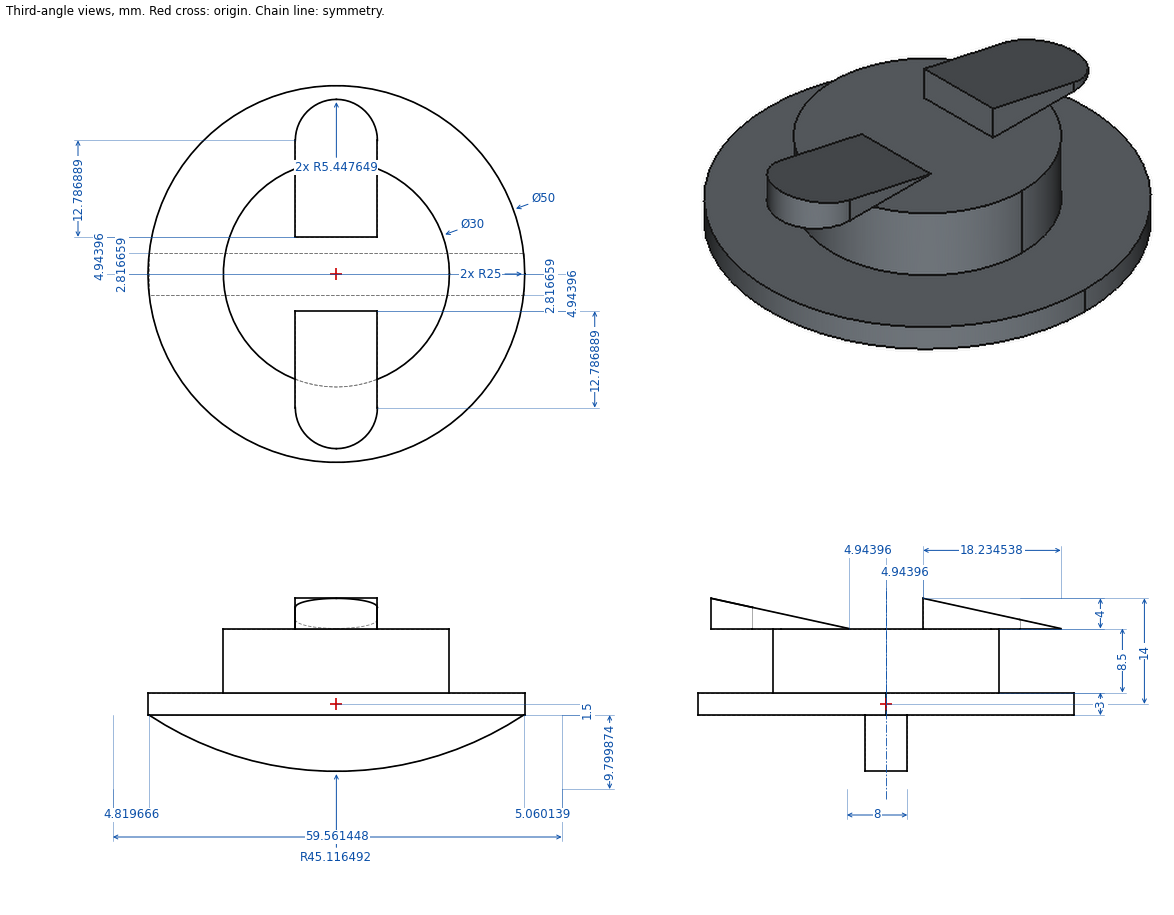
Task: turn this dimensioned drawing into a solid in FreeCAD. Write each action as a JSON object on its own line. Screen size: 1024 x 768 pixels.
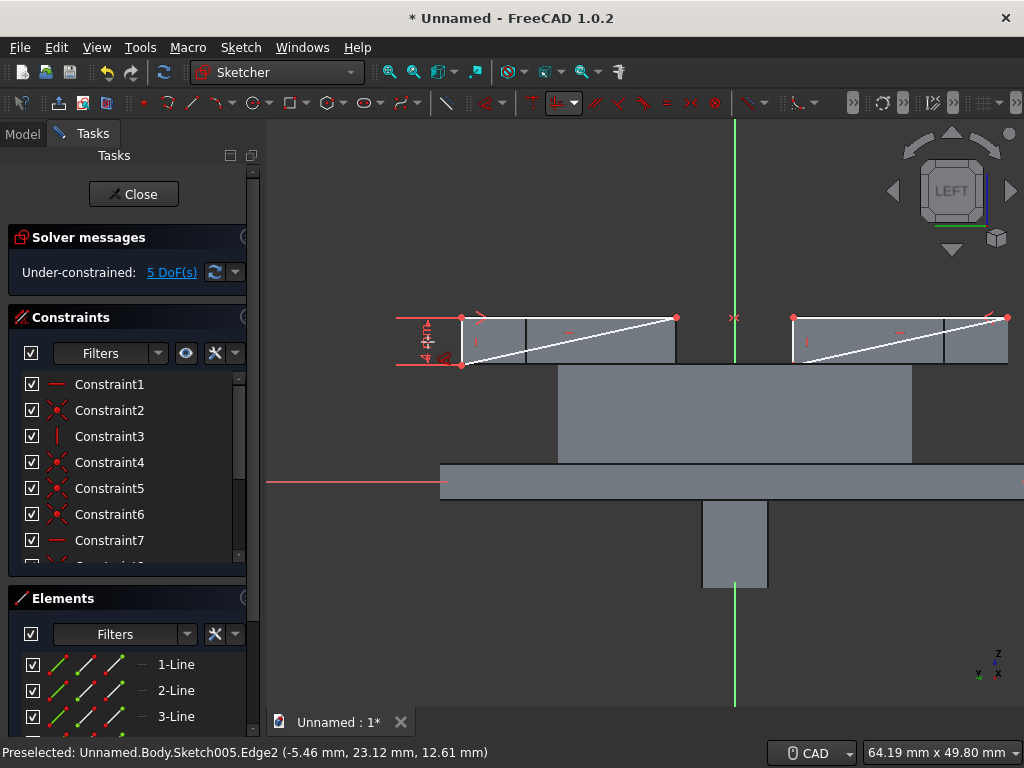
{"action": "left_click", "coordinate": [793, 332]}
{"action": "left_click", "coordinate": [827, 342]}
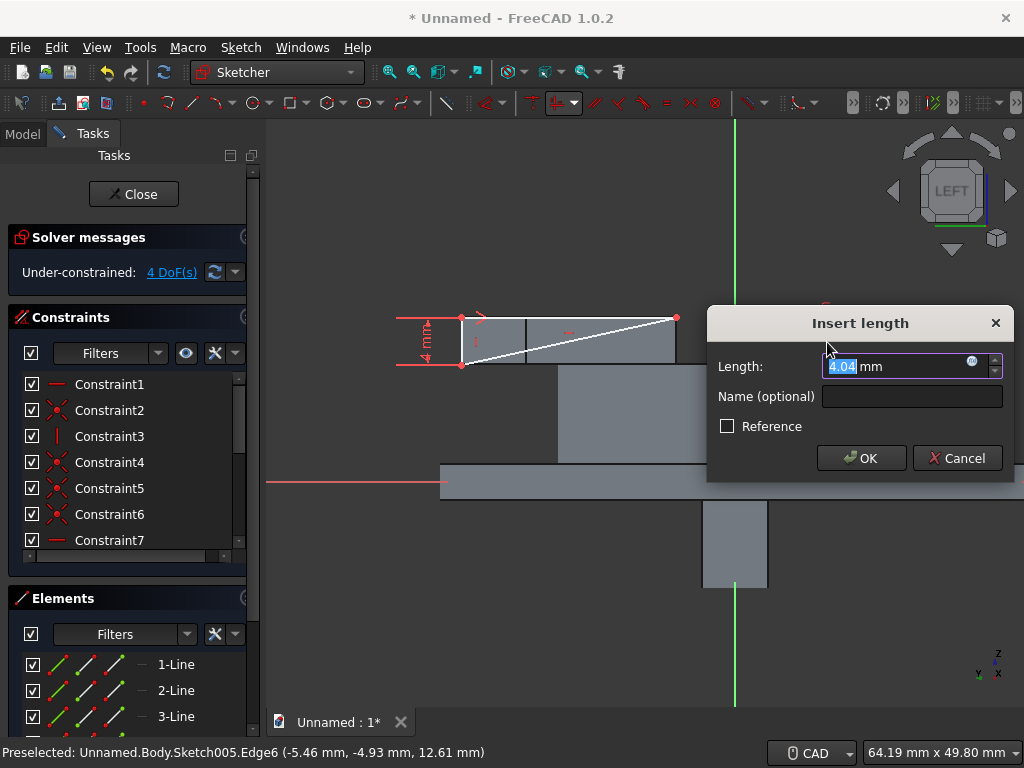
{"action": "type", "text": "4"}
{"action": "key", "text": "Return"}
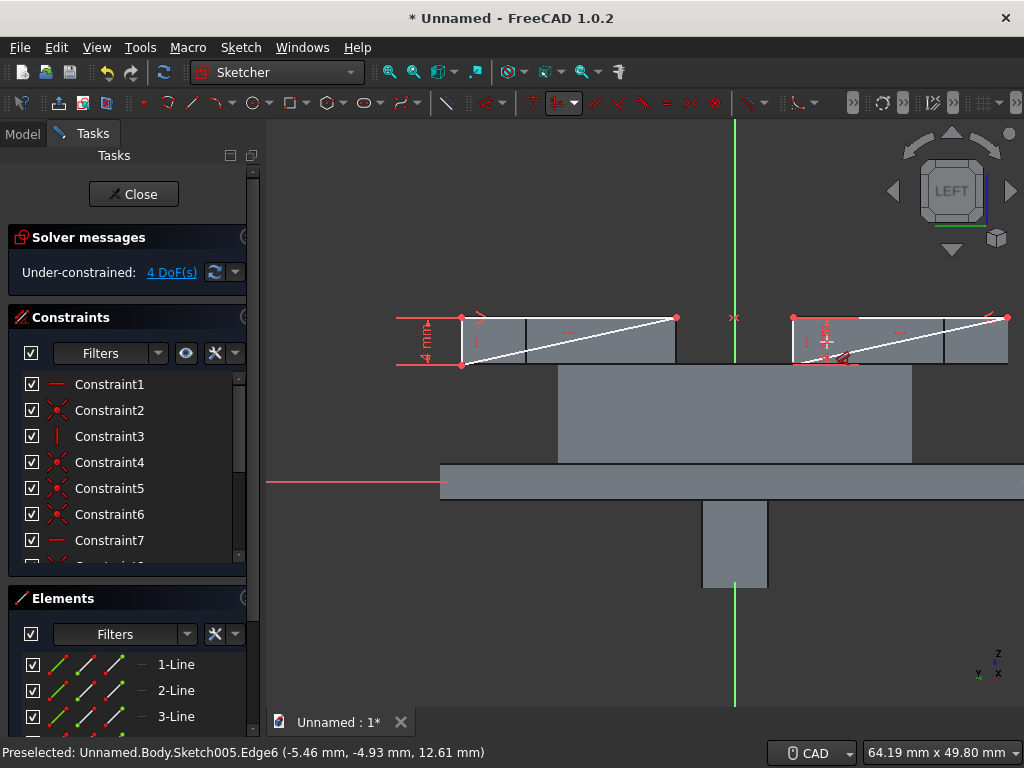
{"action": "left_click", "coordinate": [677, 318]}
{"action": "left_click", "coordinate": [643, 400]}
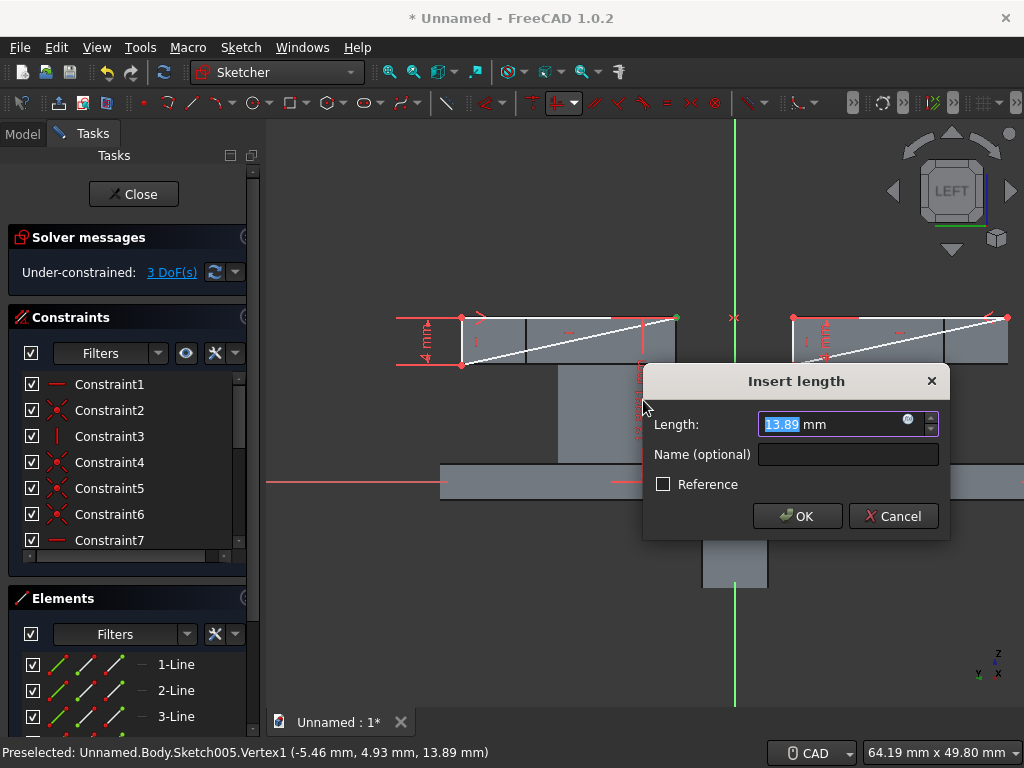
{"action": "type", "text": "14"}
{"action": "key", "text": "Return"}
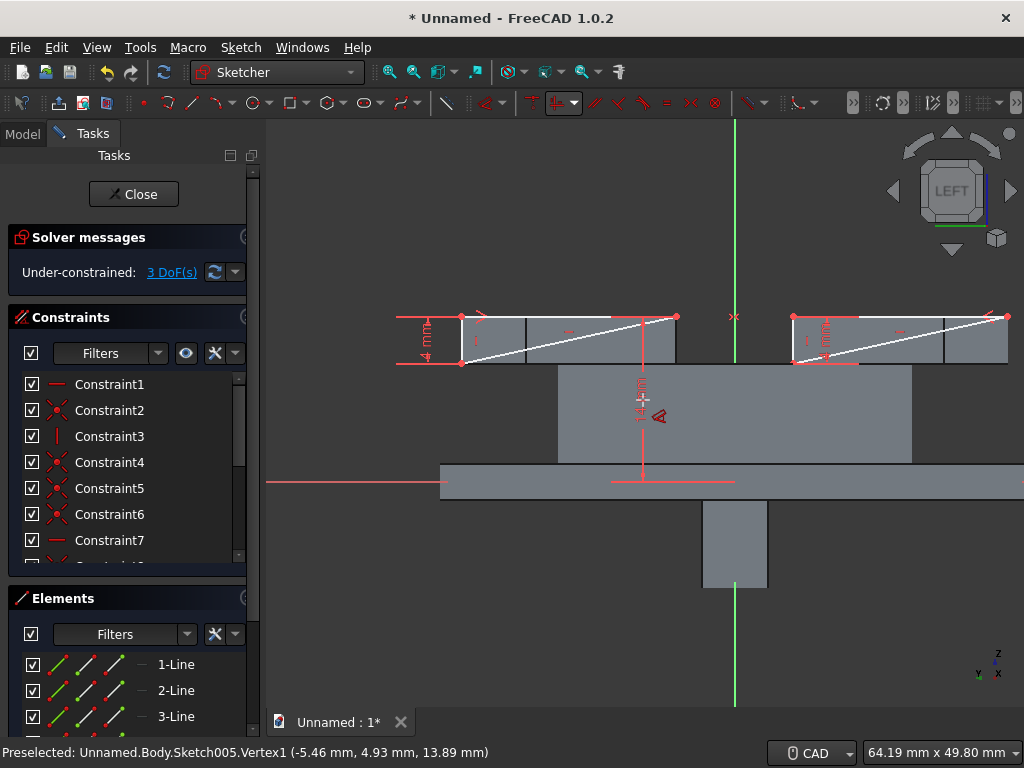
{"action": "left_click", "coordinate": [677, 317]}
{"action": "left_click", "coordinate": [706, 516]}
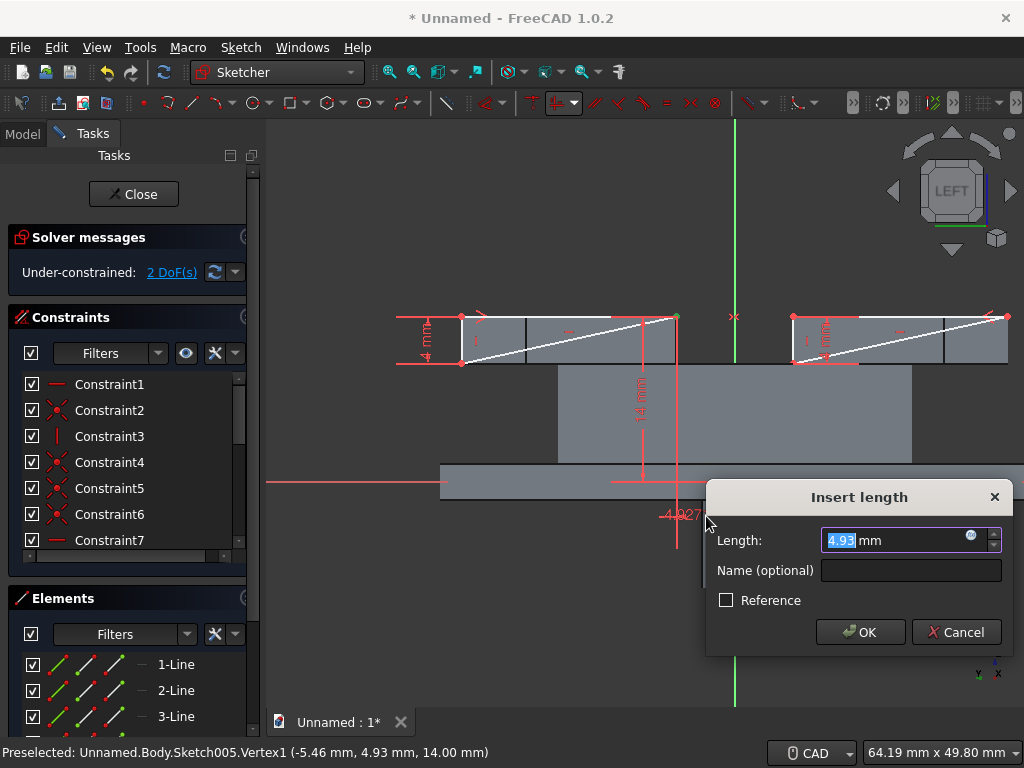
{"action": "type", "text": "4.94396"}
{"action": "key", "text": "Return"}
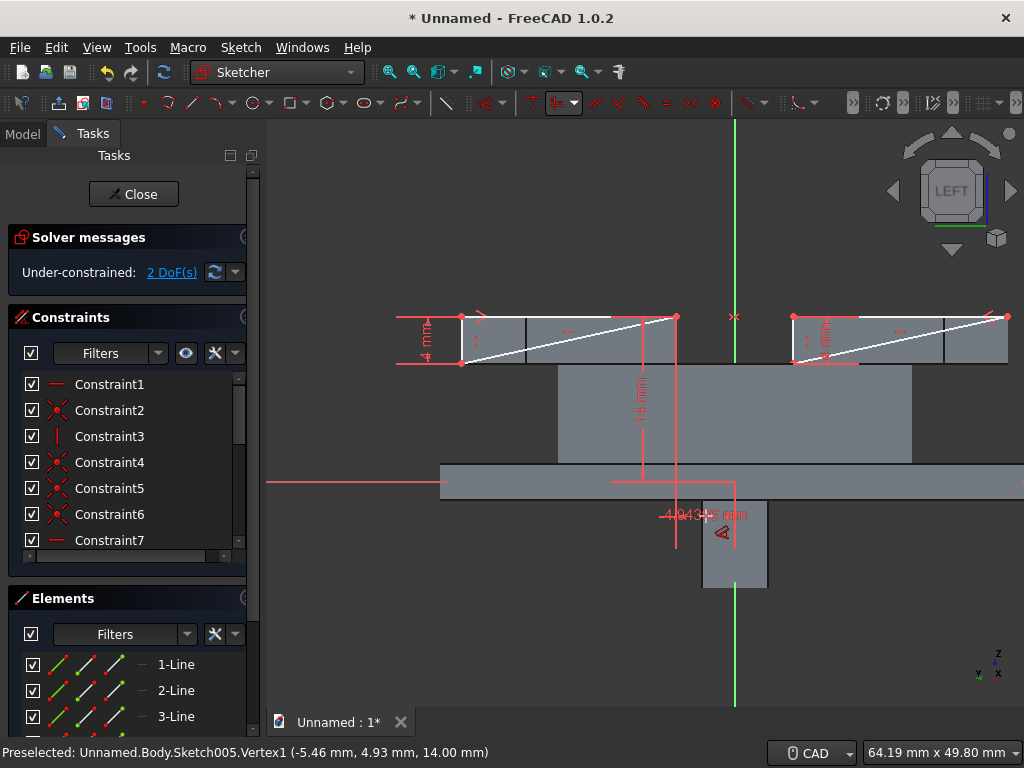
{"action": "left_click", "coordinate": [793, 364]}
{"action": "left_click", "coordinate": [777, 516]}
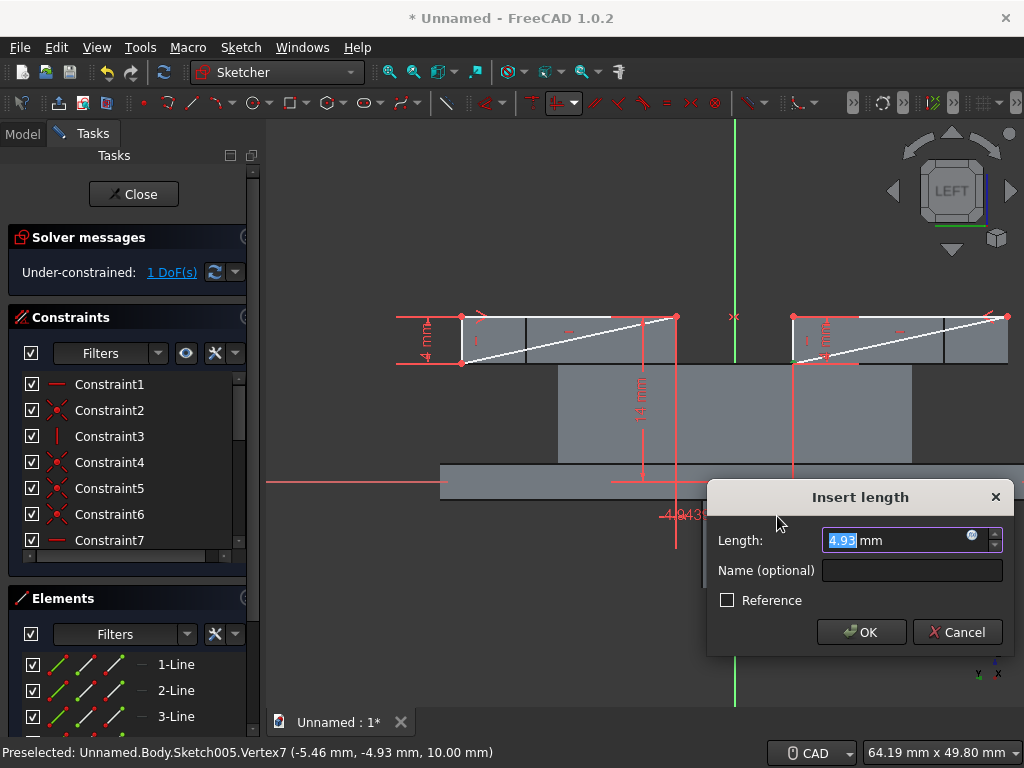
{"action": "type", "text": "4.94396"}
{"action": "key", "text": "Return"}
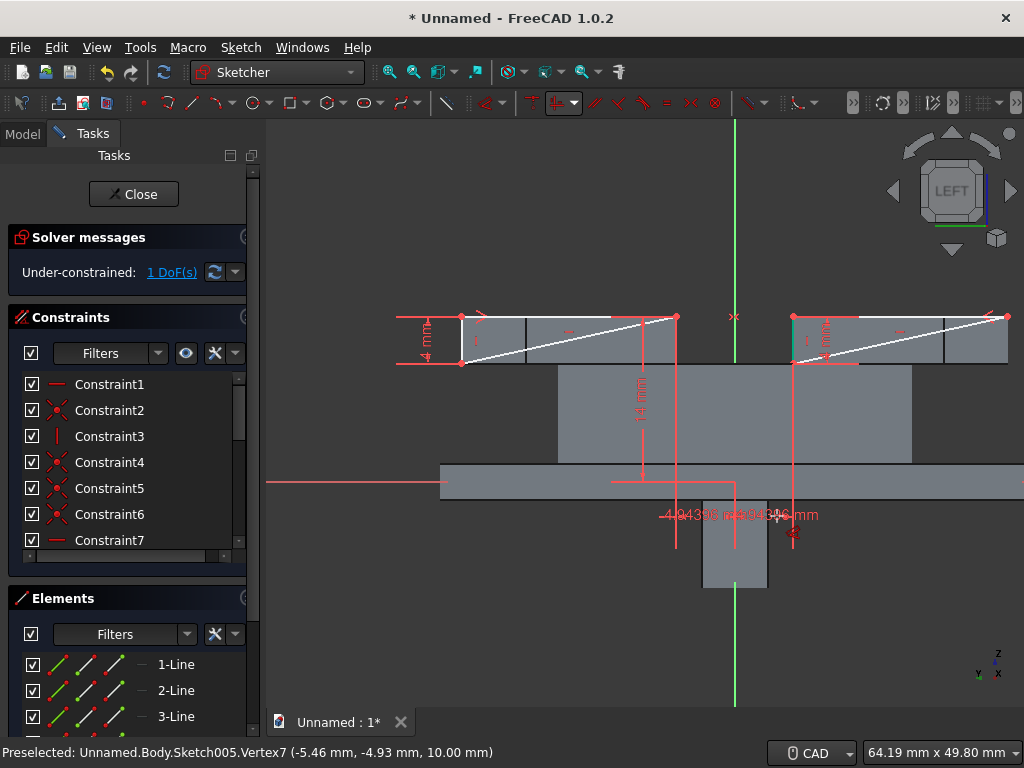
{"action": "left_click", "coordinate": [612, 317]}
{"action": "left_click", "coordinate": [569, 283]}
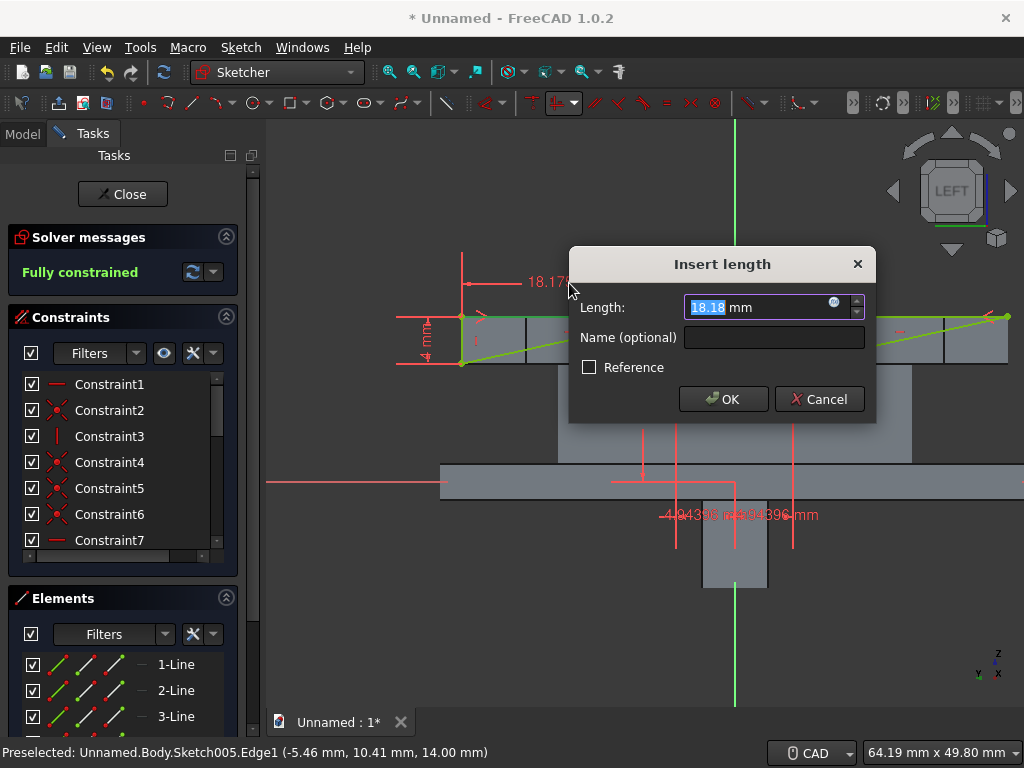
{"action": "type", "text": "18.234538"}
{"action": "key", "text": "Return"}
{"action": "key", "text": "Escape"}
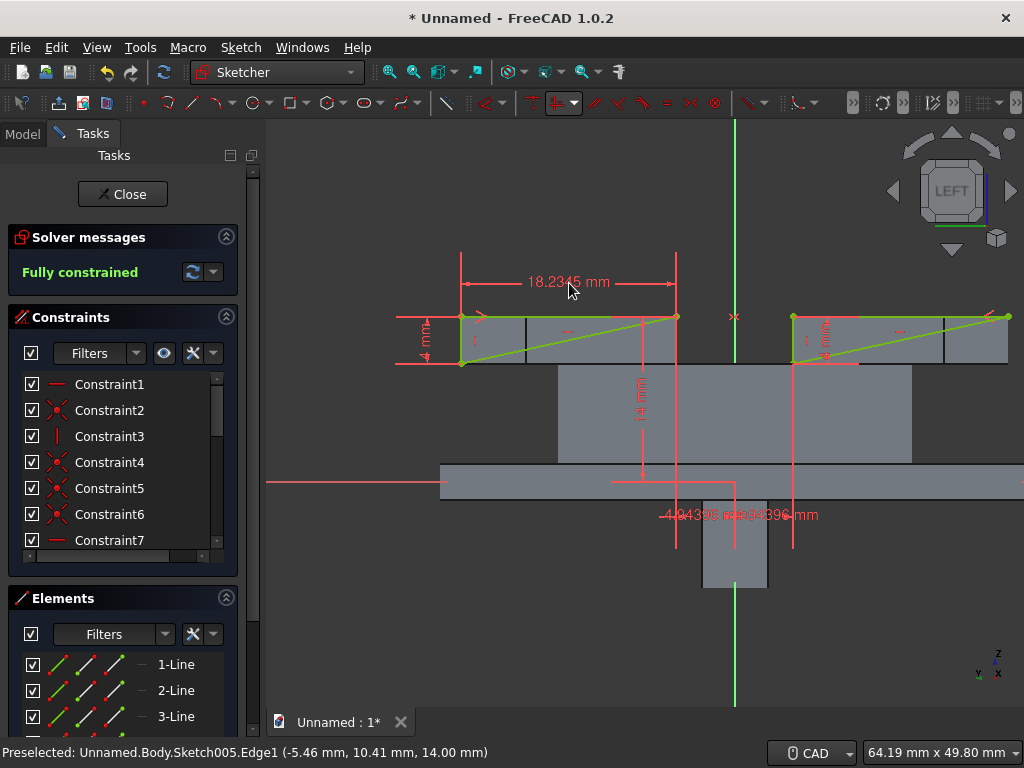
{"action": "left_click", "coordinate": [123, 194]}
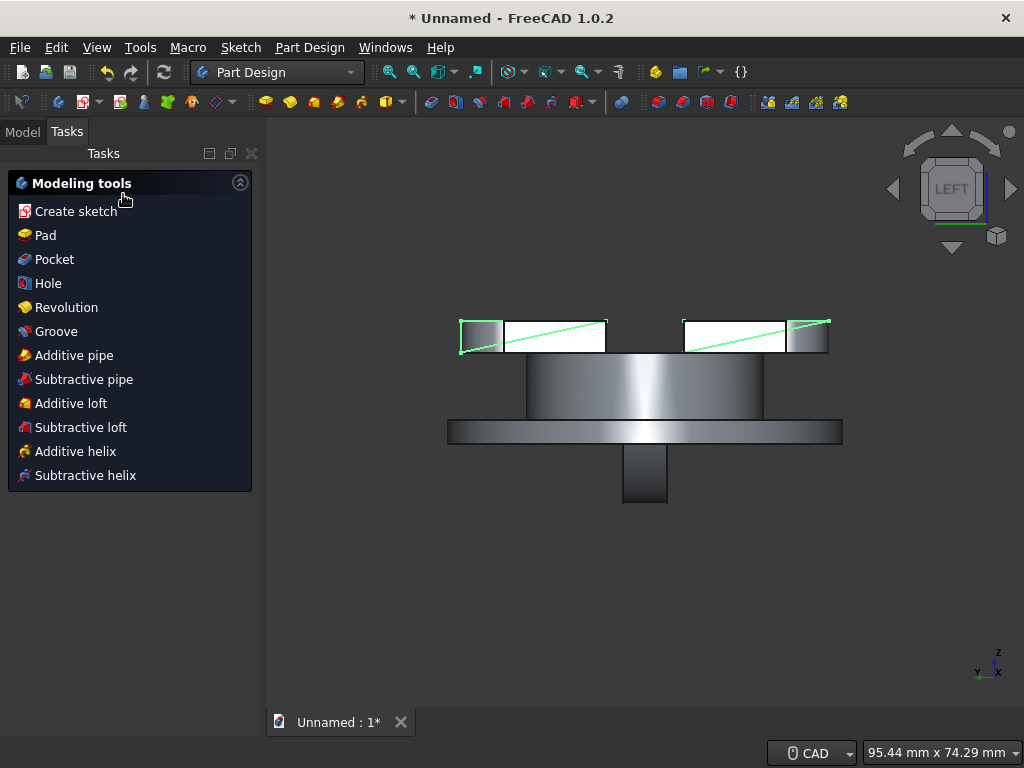
{"action": "left_click", "coordinate": [432, 102]}